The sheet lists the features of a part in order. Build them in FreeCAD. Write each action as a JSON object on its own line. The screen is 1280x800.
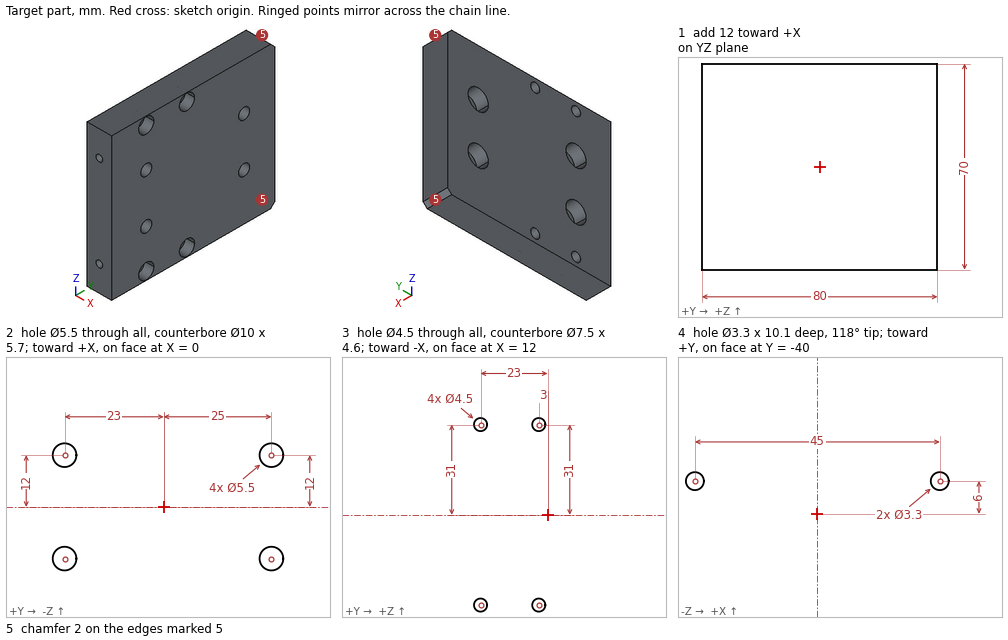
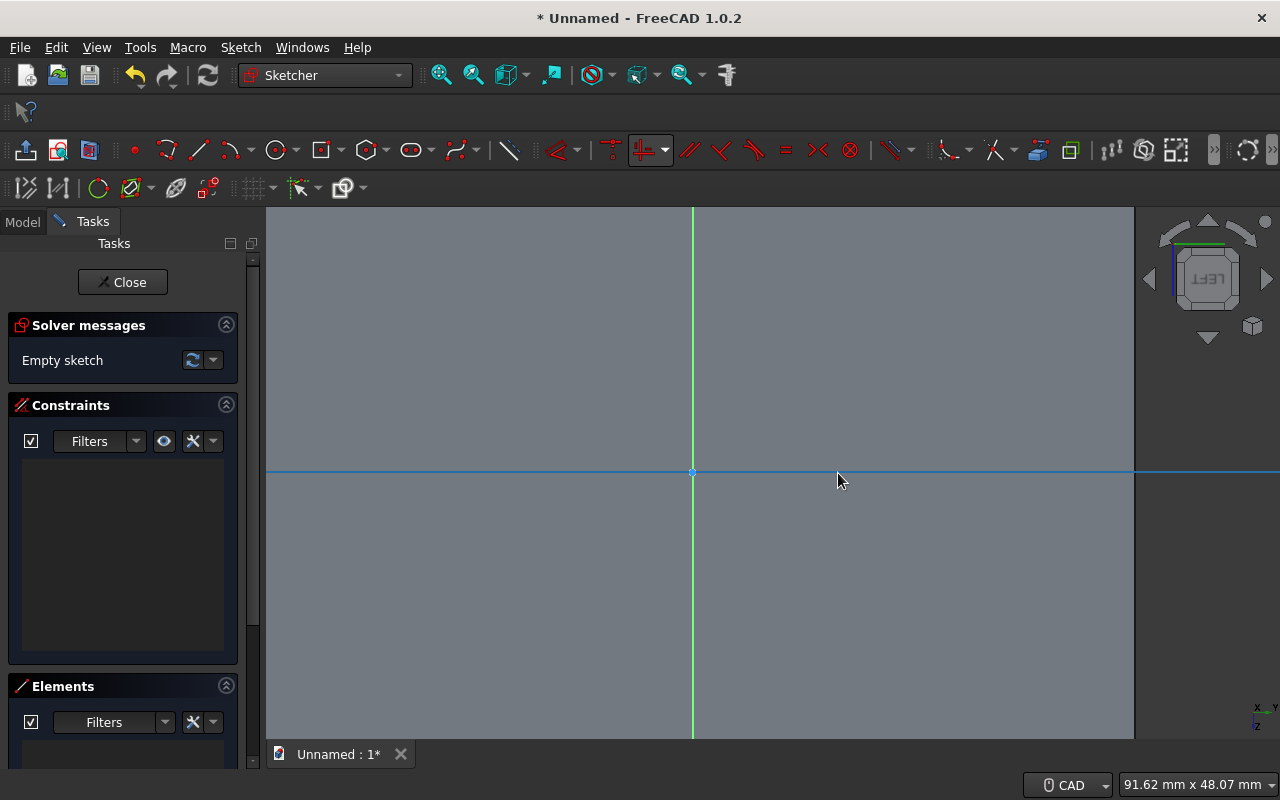
{"action": "left_click", "coordinate": [276, 150]}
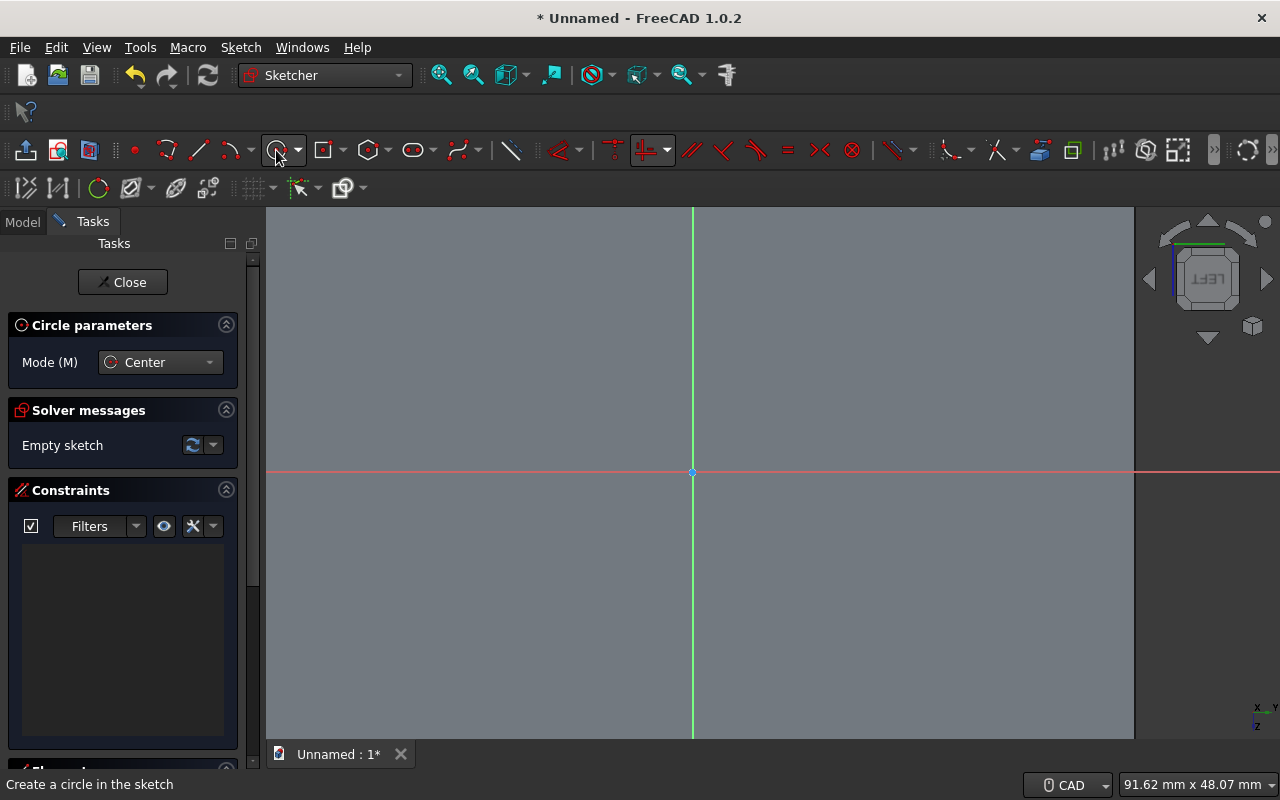
{"action": "left_click", "coordinate": [969, 340]}
{"action": "left_click", "coordinate": [991, 318]}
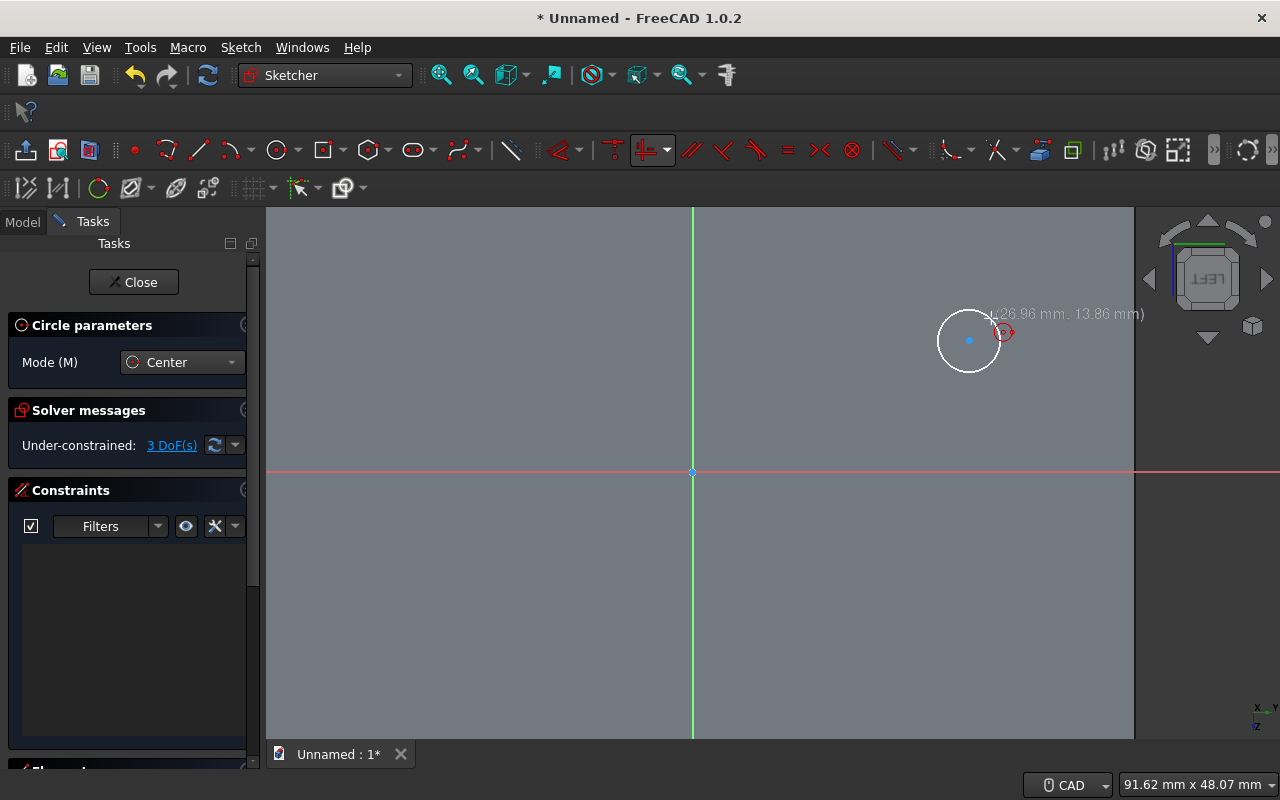
{"action": "left_click", "coordinate": [438, 340]}
{"action": "left_click", "coordinate": [460, 318]}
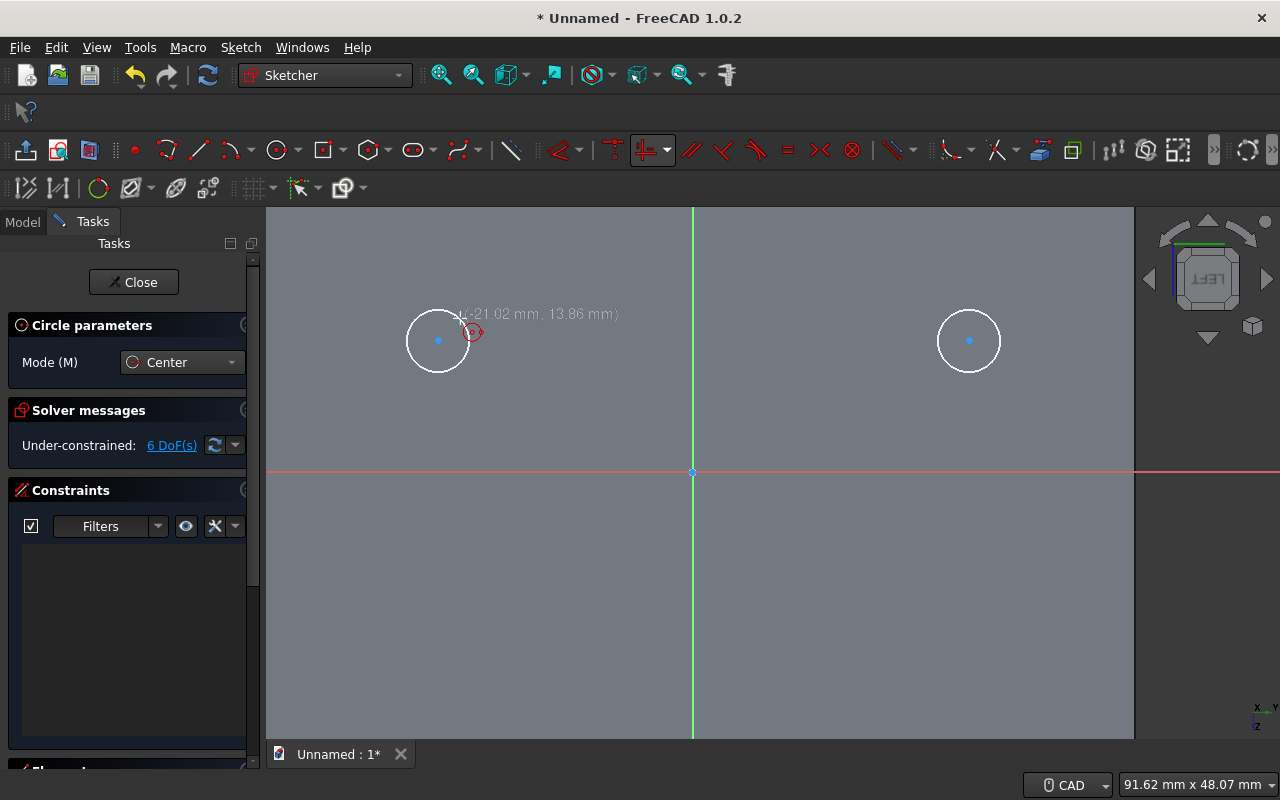
{"action": "left_click", "coordinate": [438, 605]}
{"action": "left_click", "coordinate": [460, 584]}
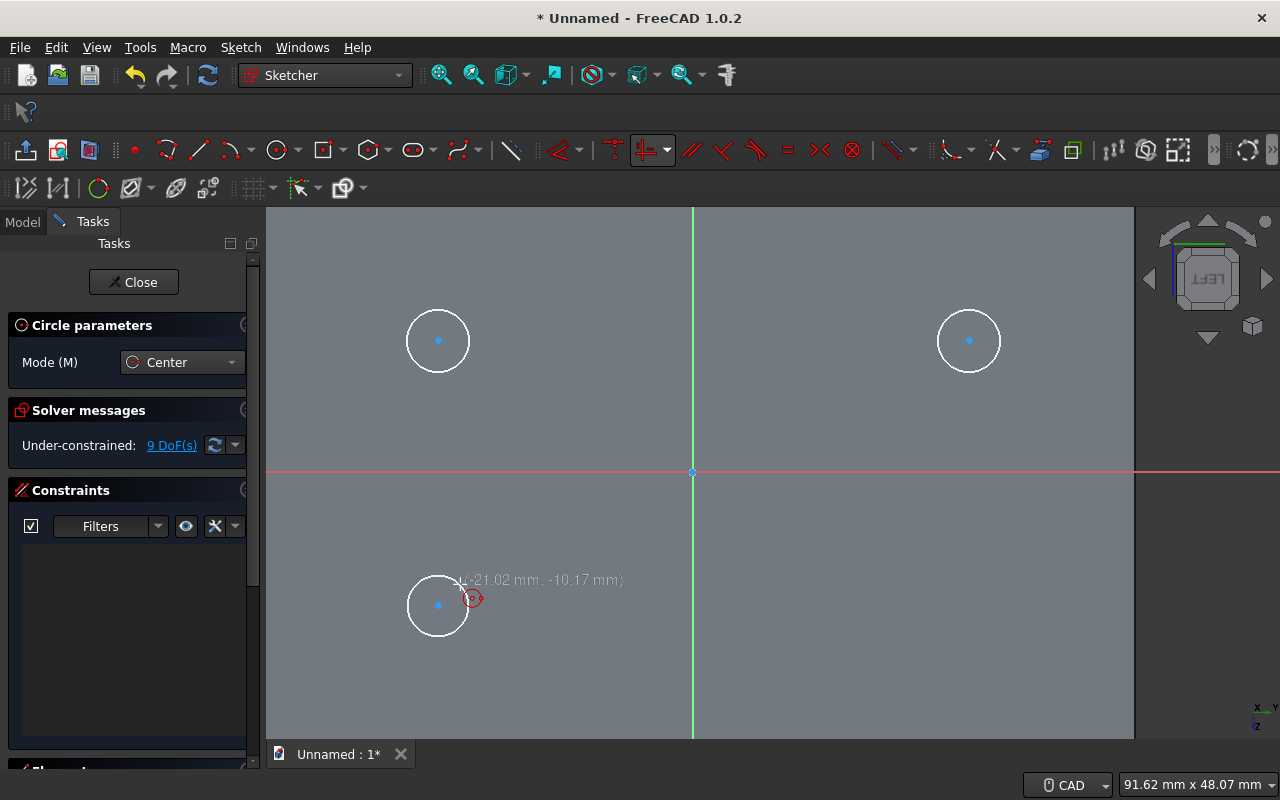
{"action": "left_click", "coordinate": [969, 605]}
{"action": "left_click", "coordinate": [991, 584]}
{"action": "key", "text": "Escape"}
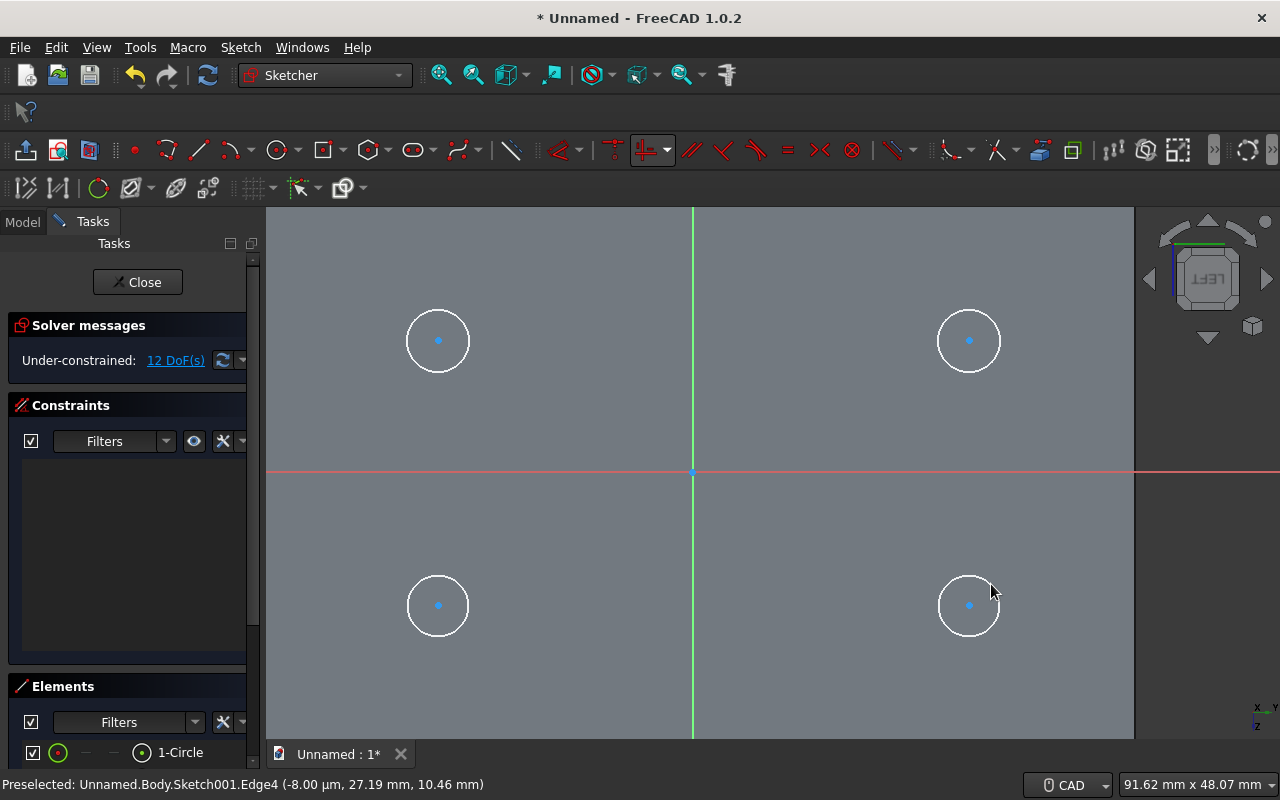
{"action": "left_click", "coordinate": [991, 319]}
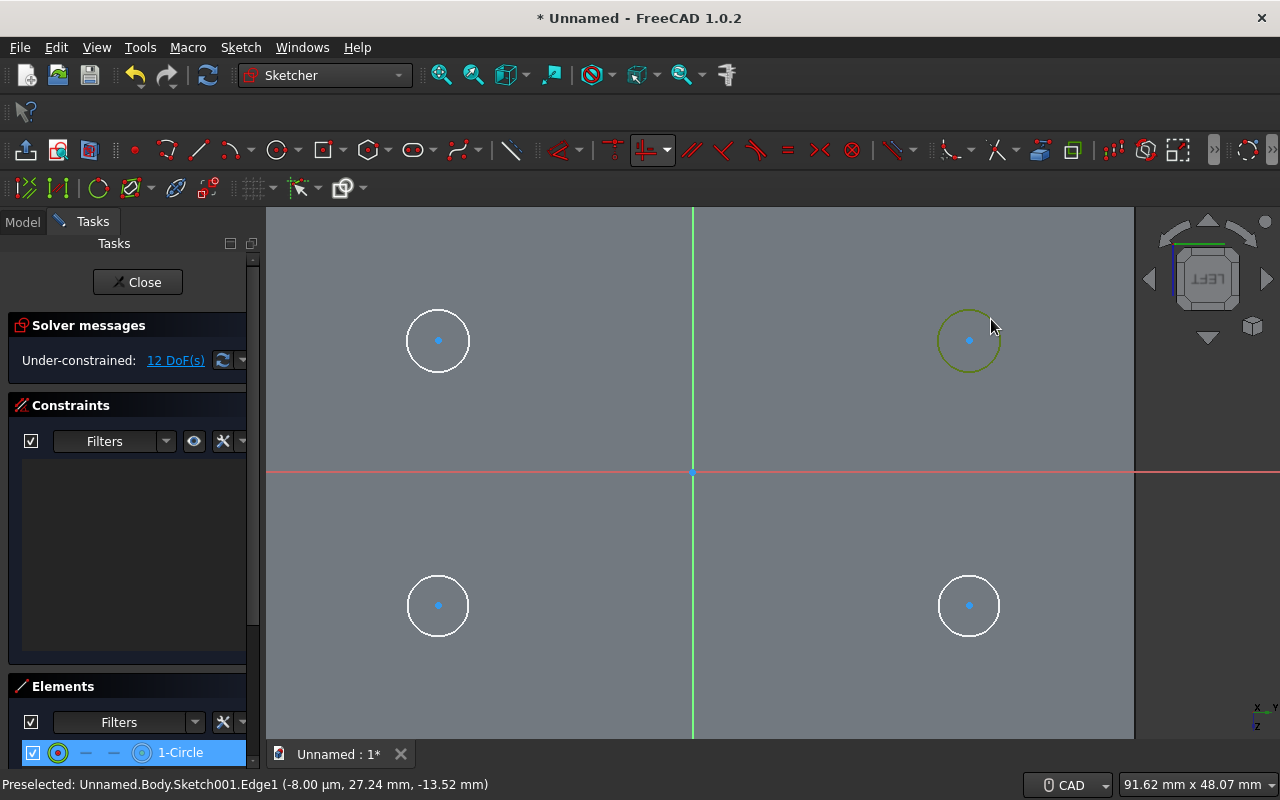
{"action": "left_click", "coordinate": [460, 319]}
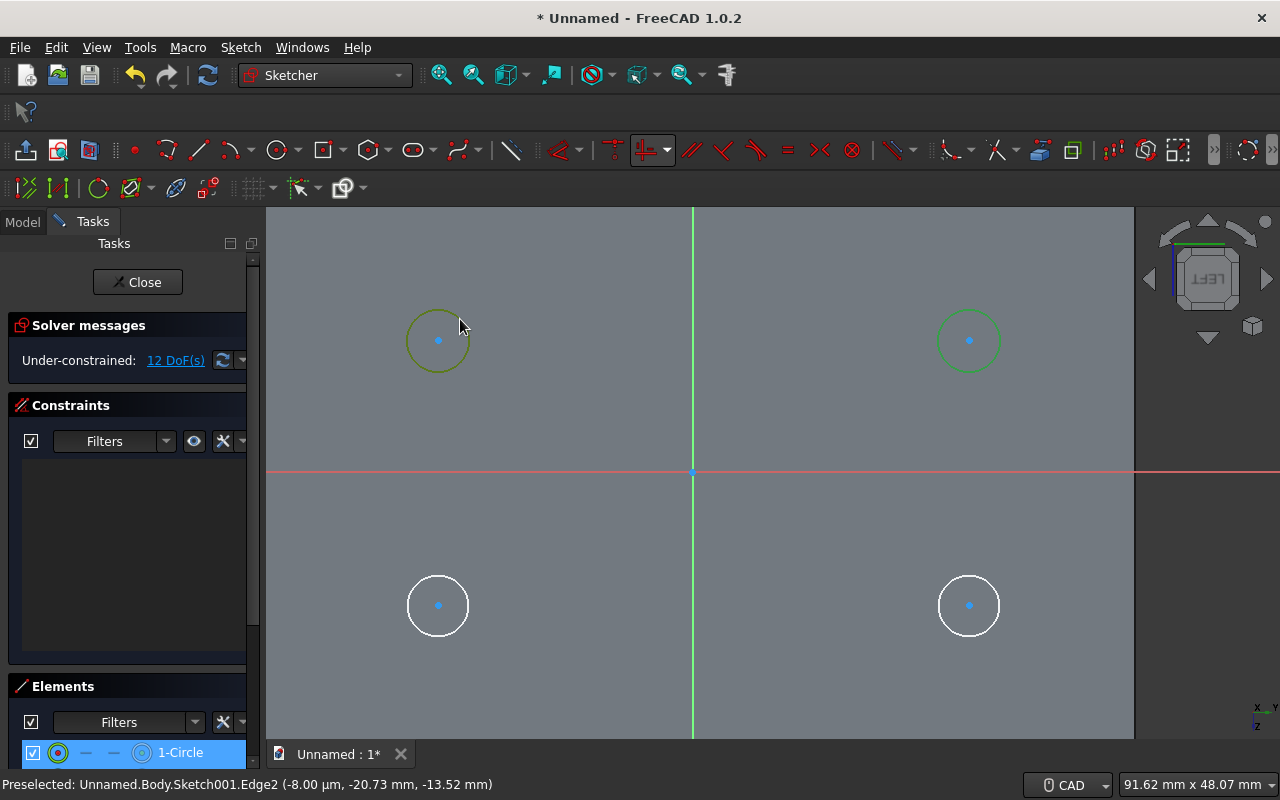
{"action": "left_click", "coordinate": [459, 584]}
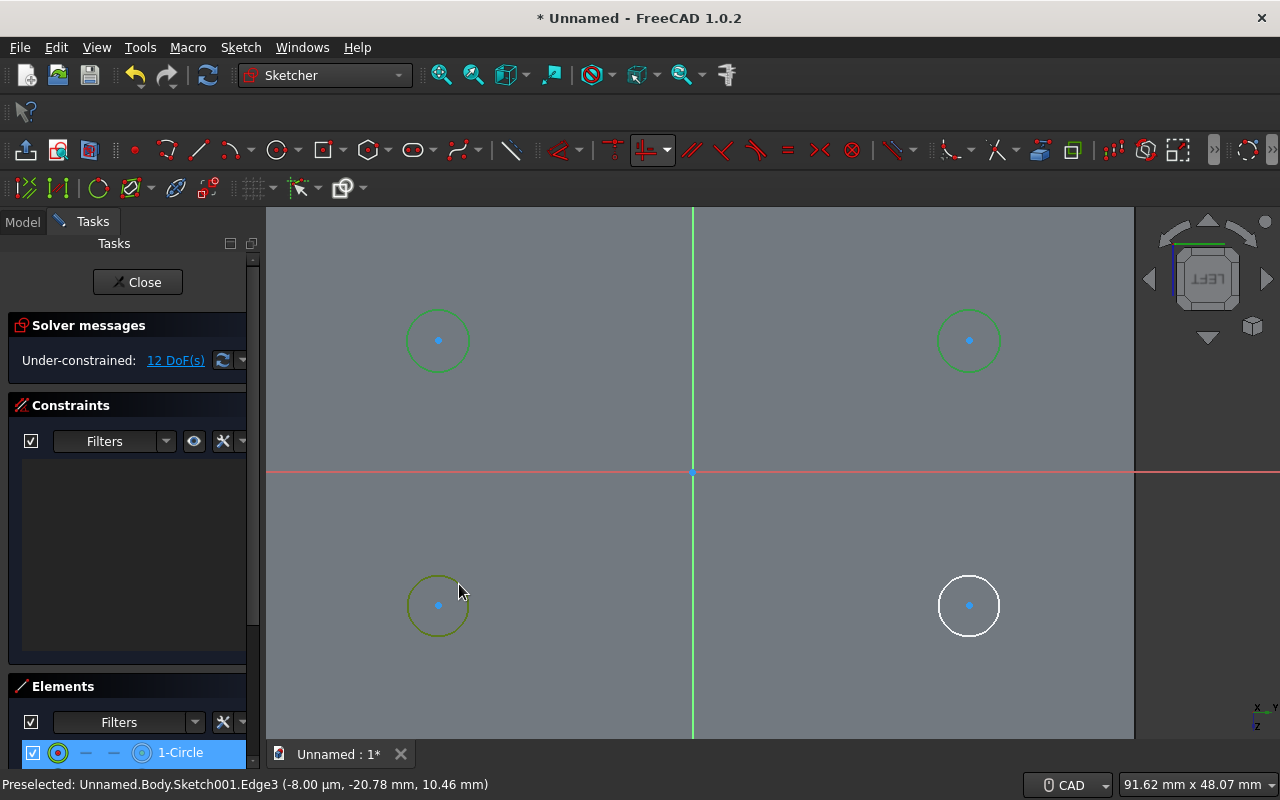
{"action": "left_click", "coordinate": [990, 584]}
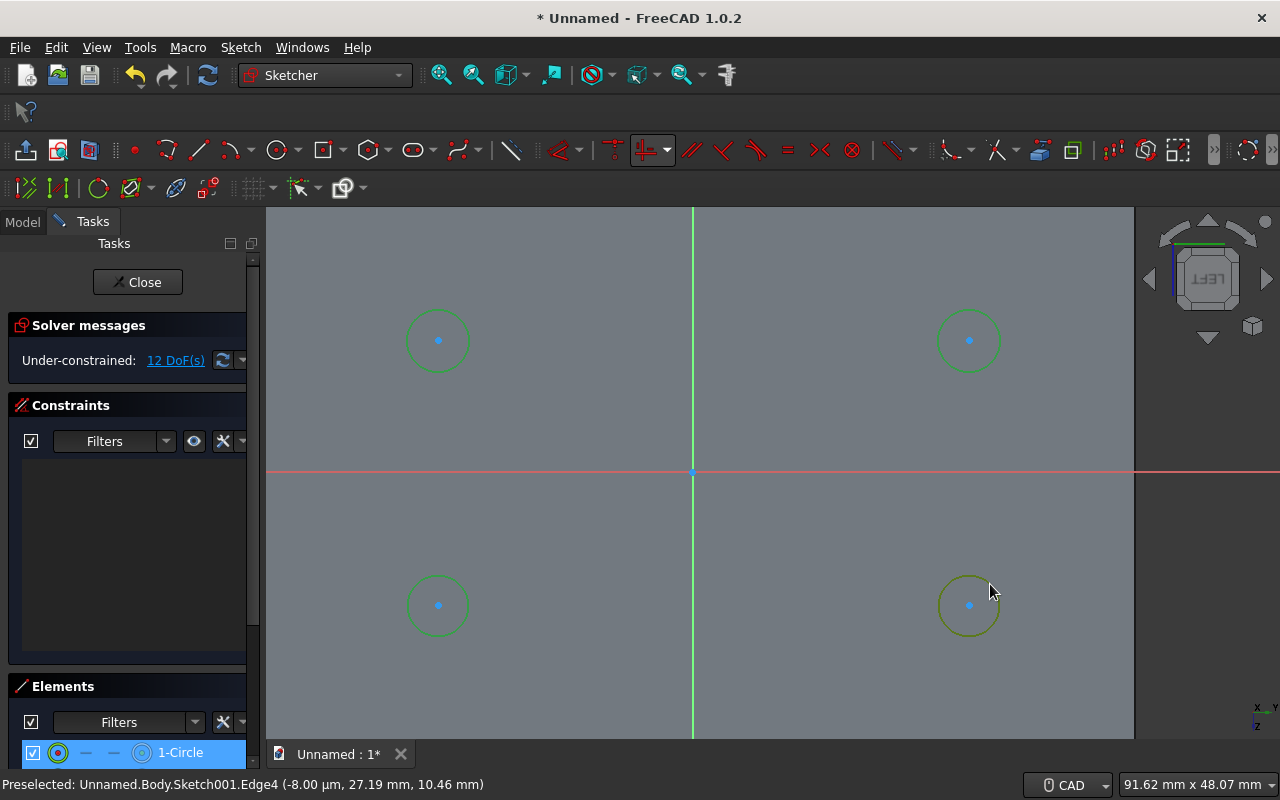
{"action": "left_click", "coordinate": [788, 150]}